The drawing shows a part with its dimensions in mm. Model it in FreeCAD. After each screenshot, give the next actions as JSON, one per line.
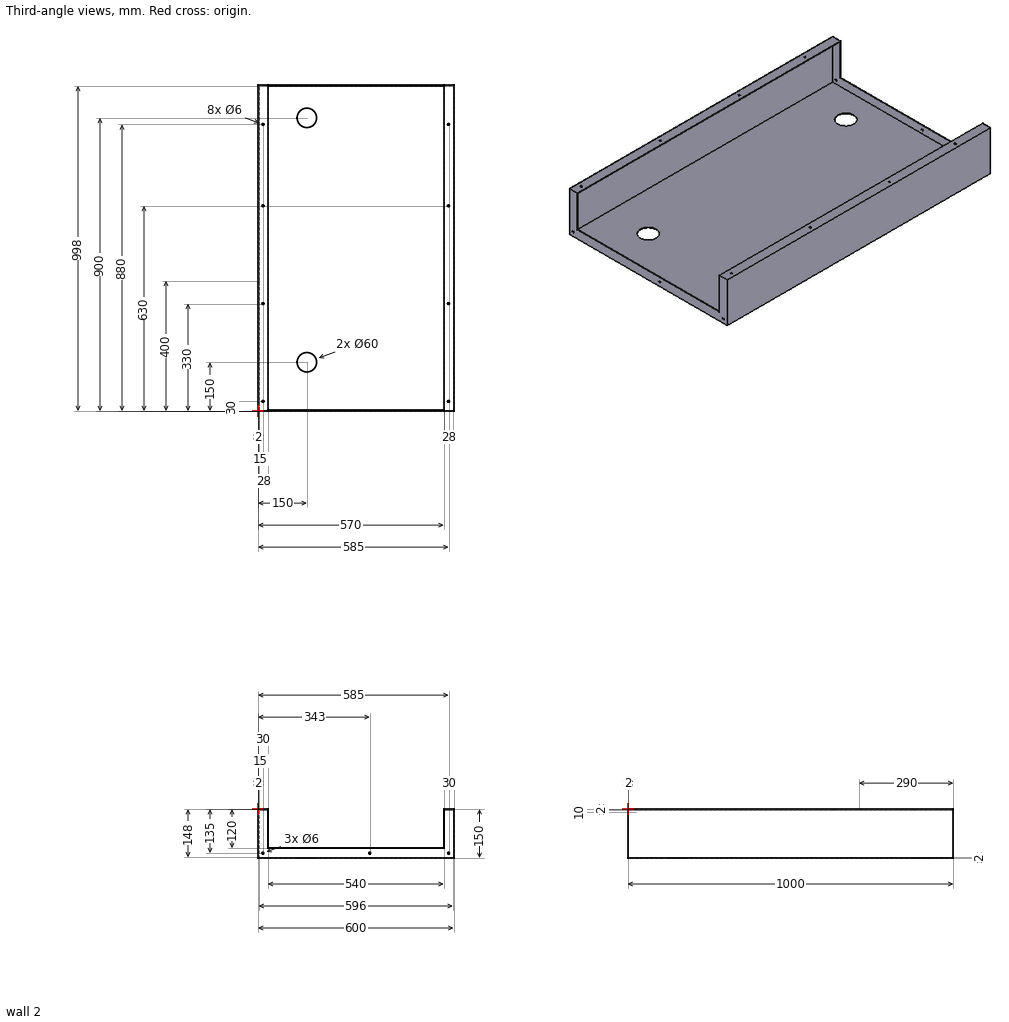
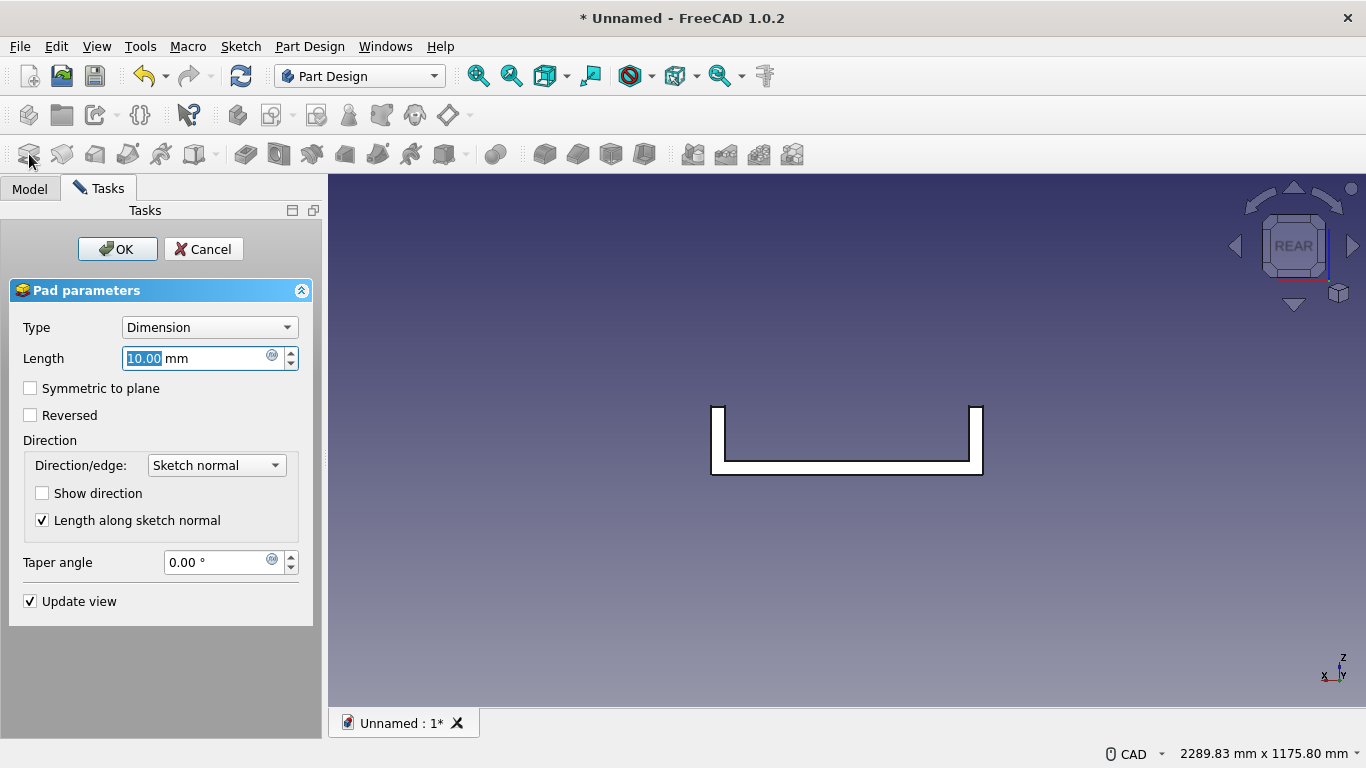
{"action": "type", "text": "2"}
{"action": "key", "text": "Tab"}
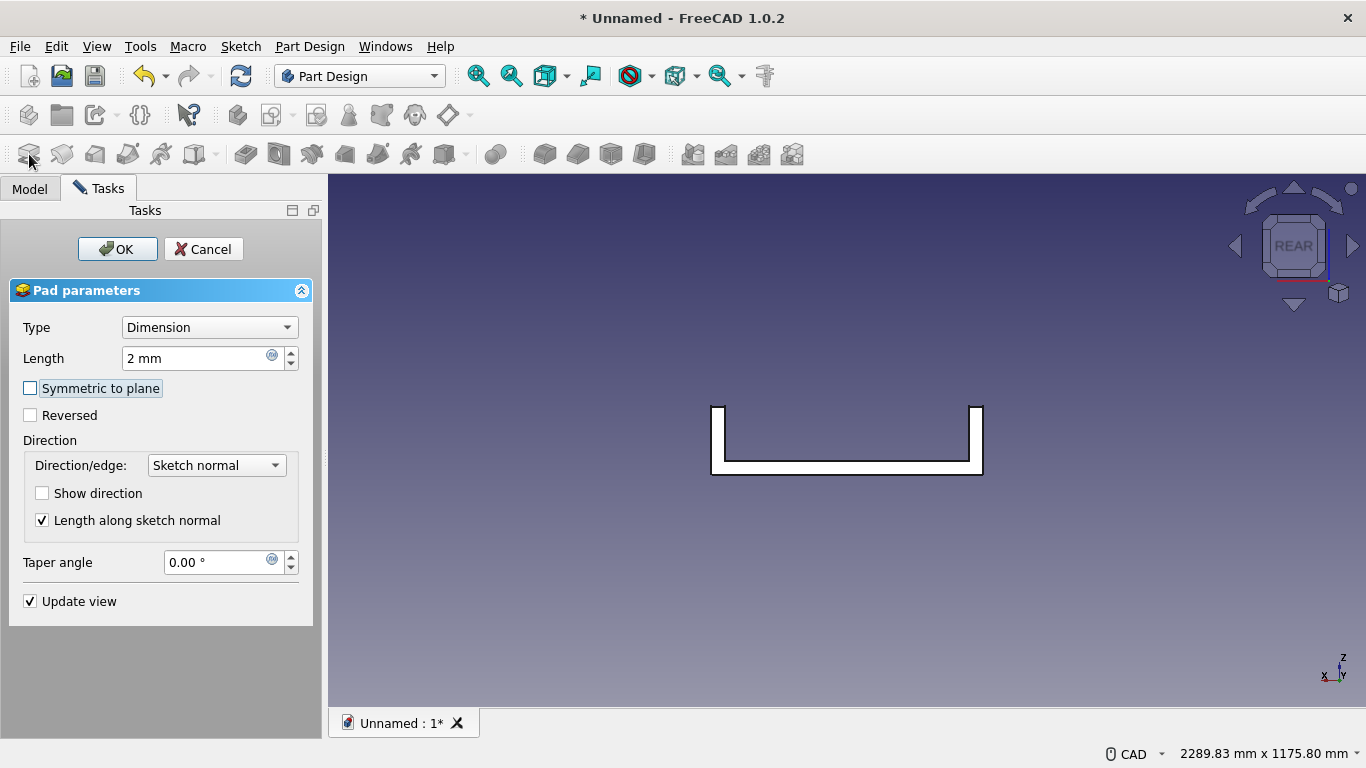
{"action": "left_click", "coordinate": [31, 415]}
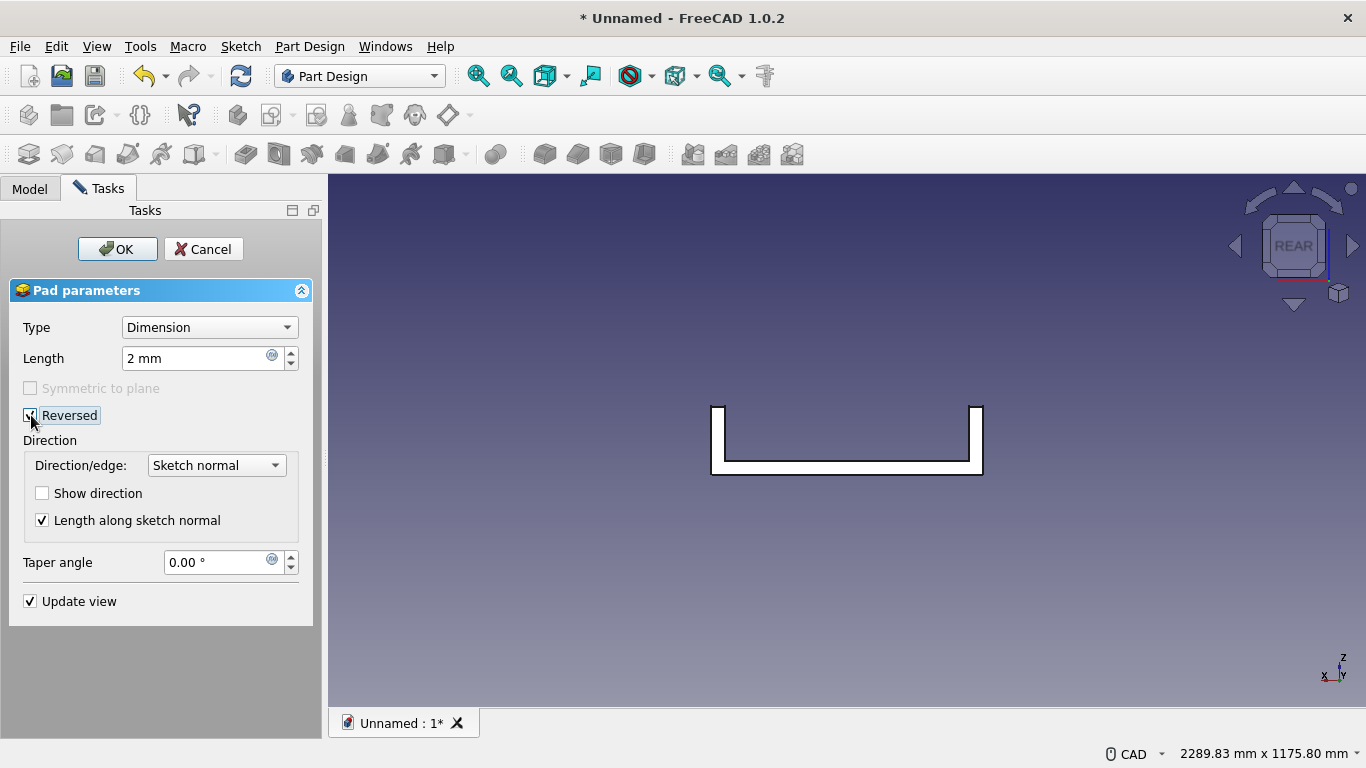
{"action": "left_click", "coordinate": [118, 249]}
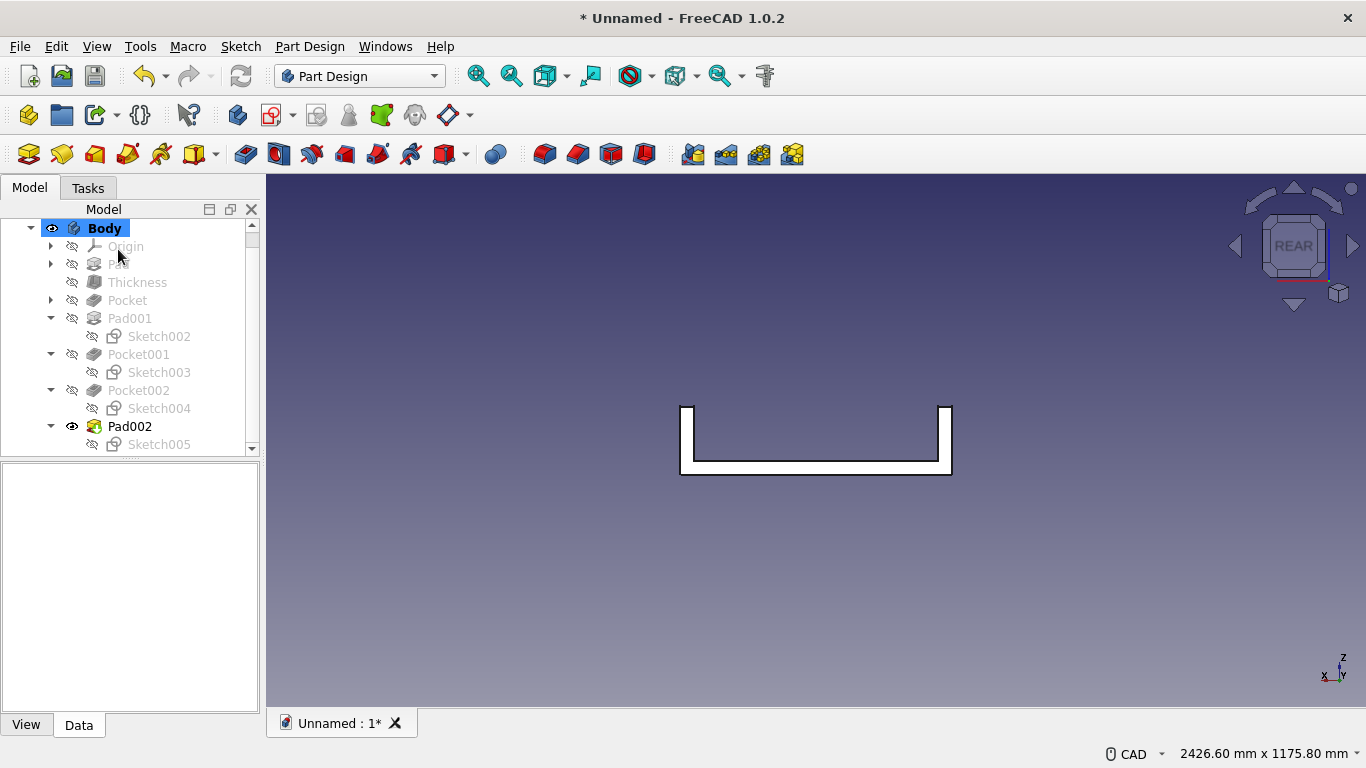
{"action": "left_click", "coordinate": [479, 76]}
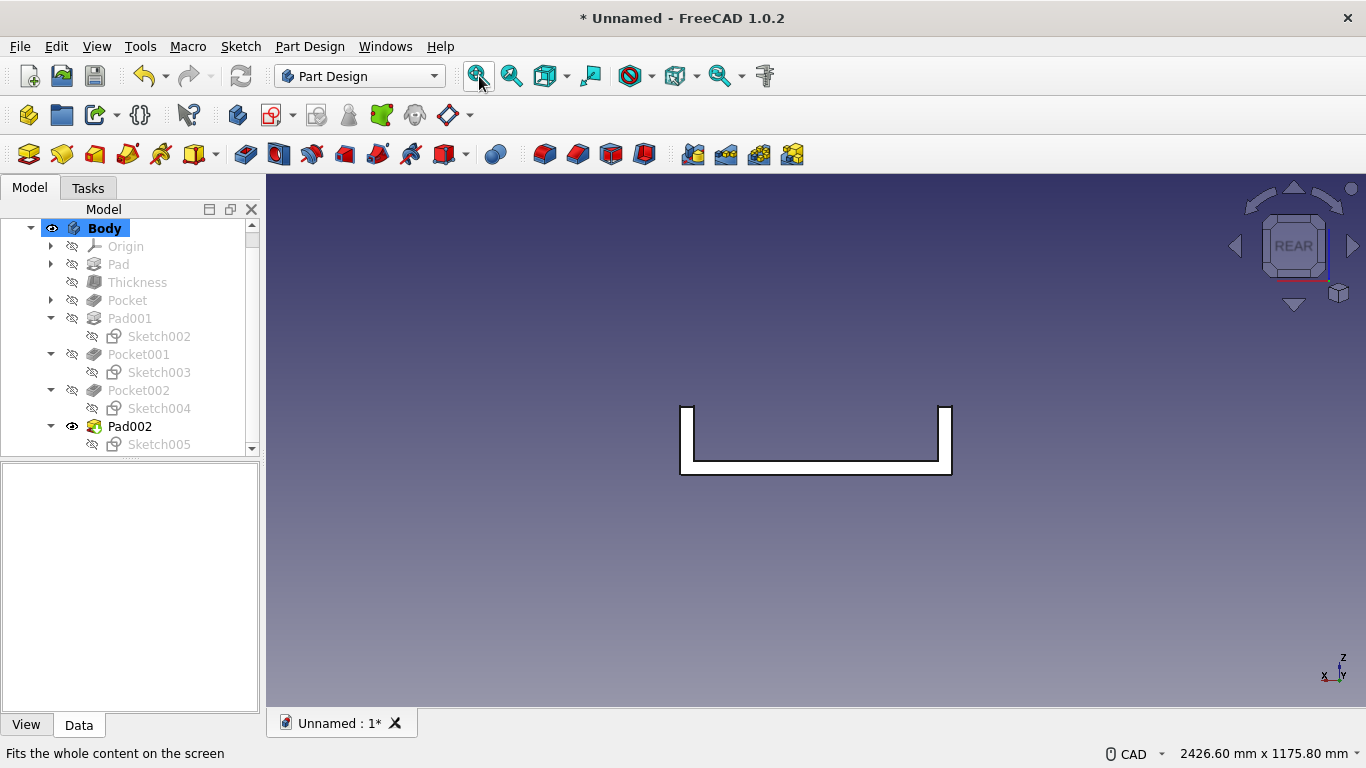
{"action": "scroll", "coordinate": [699, 469], "scroll_direction": "up", "scroll_amount": 5}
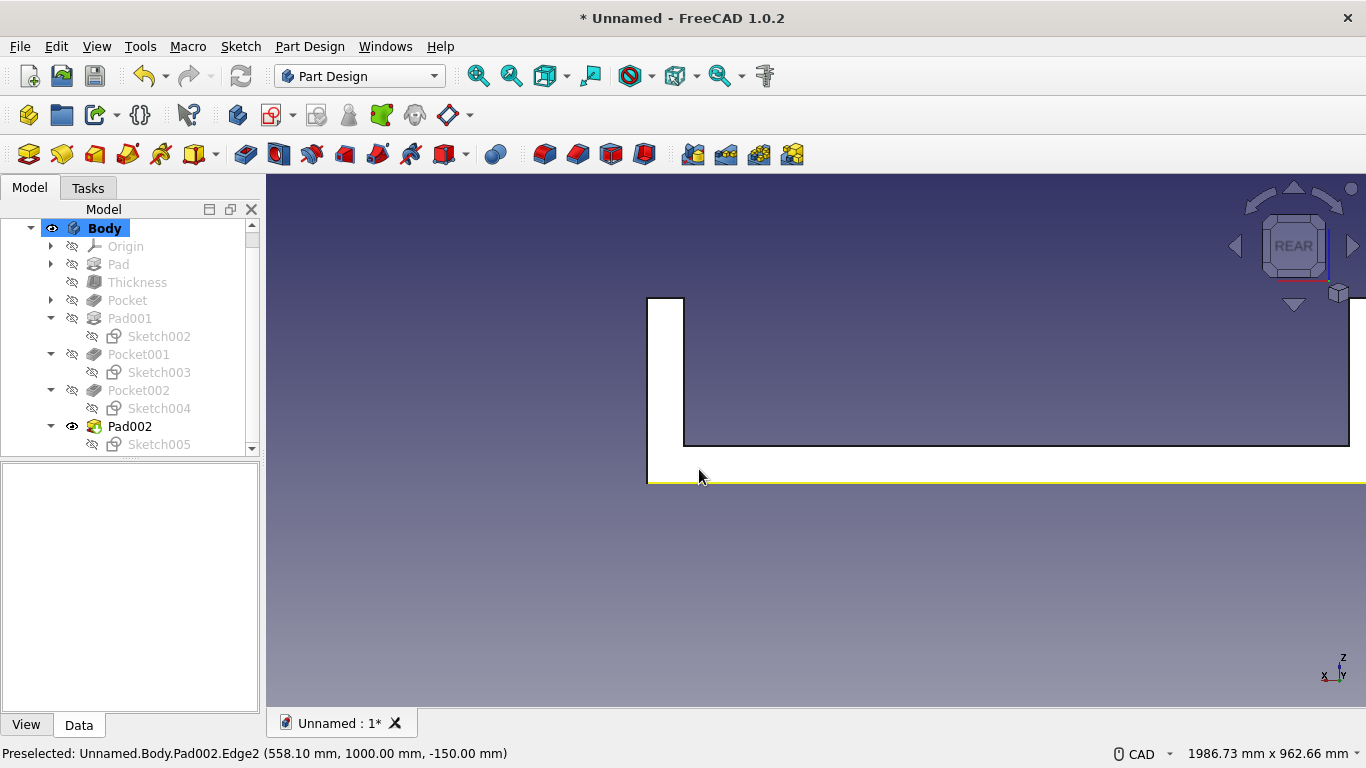
{"action": "left_click", "coordinate": [700, 469]}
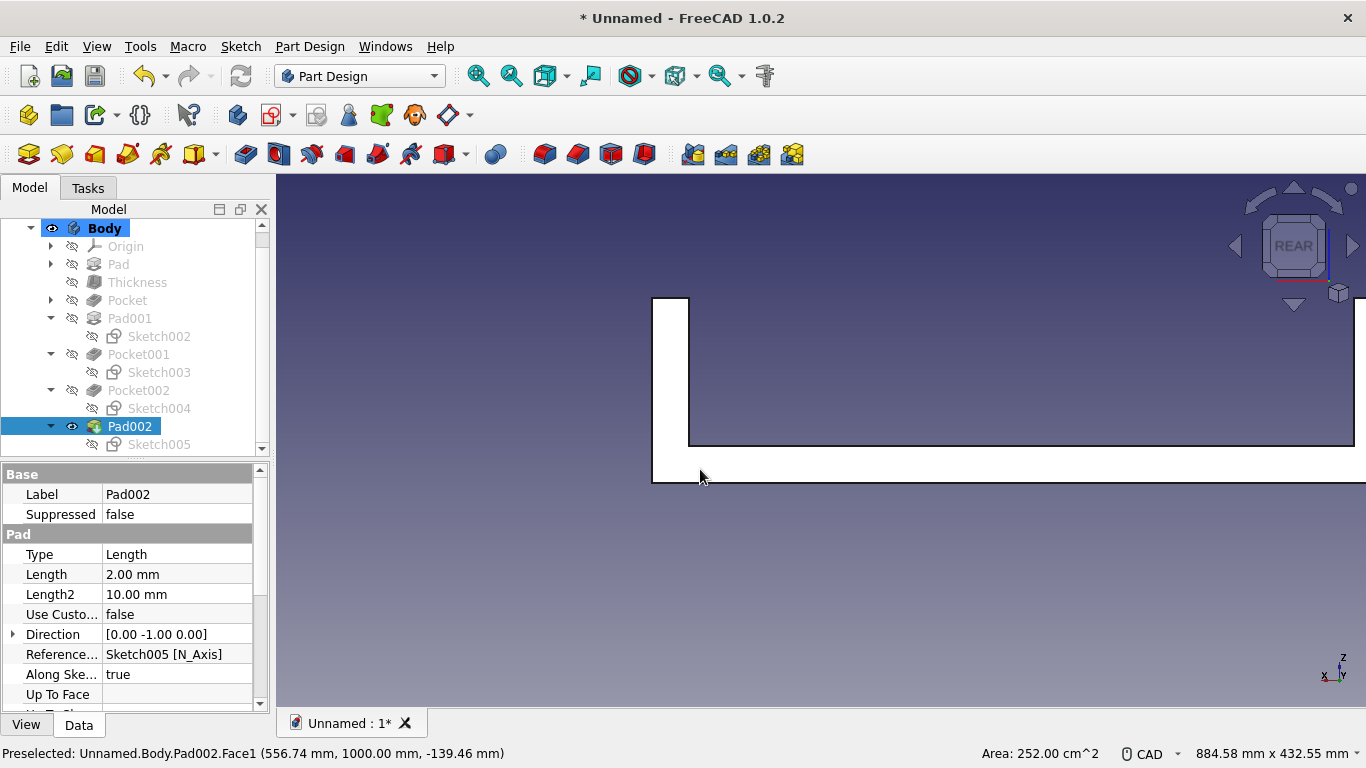
{"action": "left_click", "coordinate": [270, 116]}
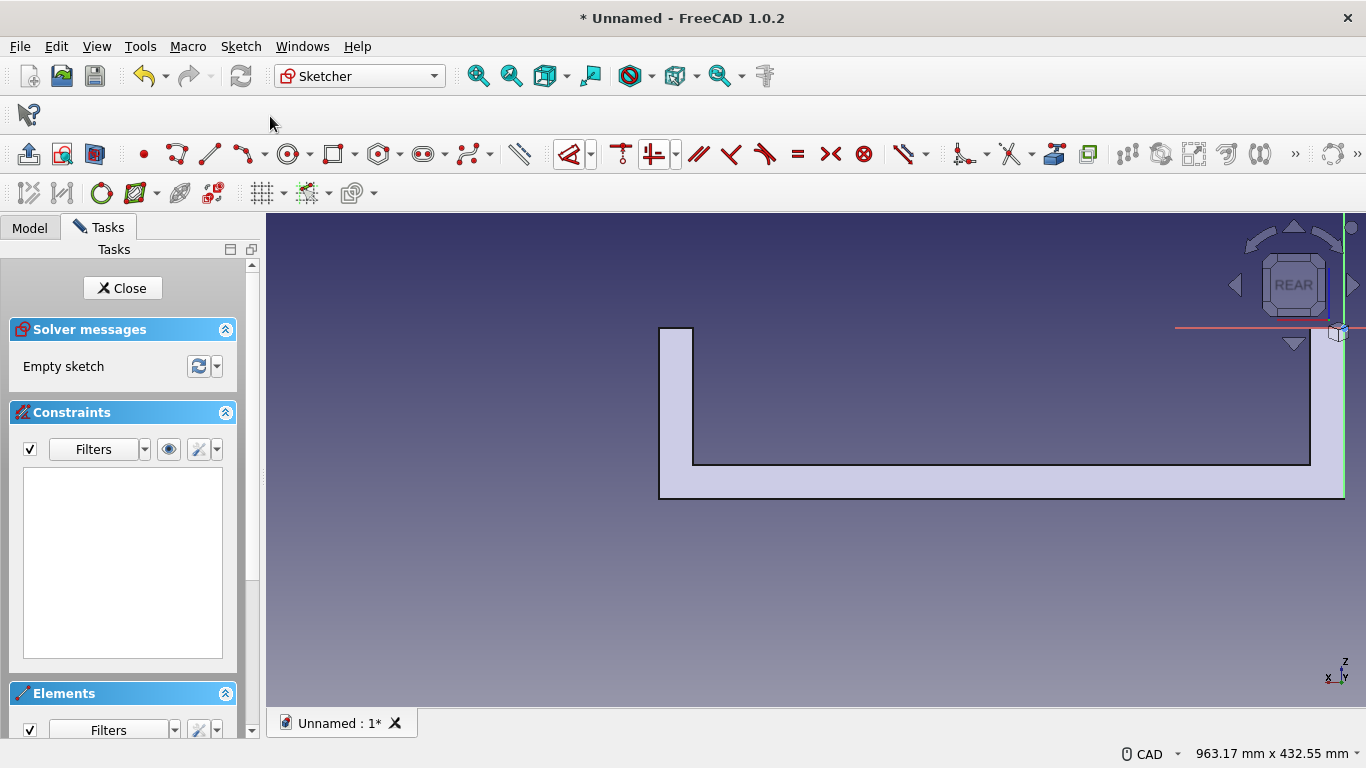
{"action": "scroll", "coordinate": [294, 679], "scroll_direction": "down", "scroll_amount": 1}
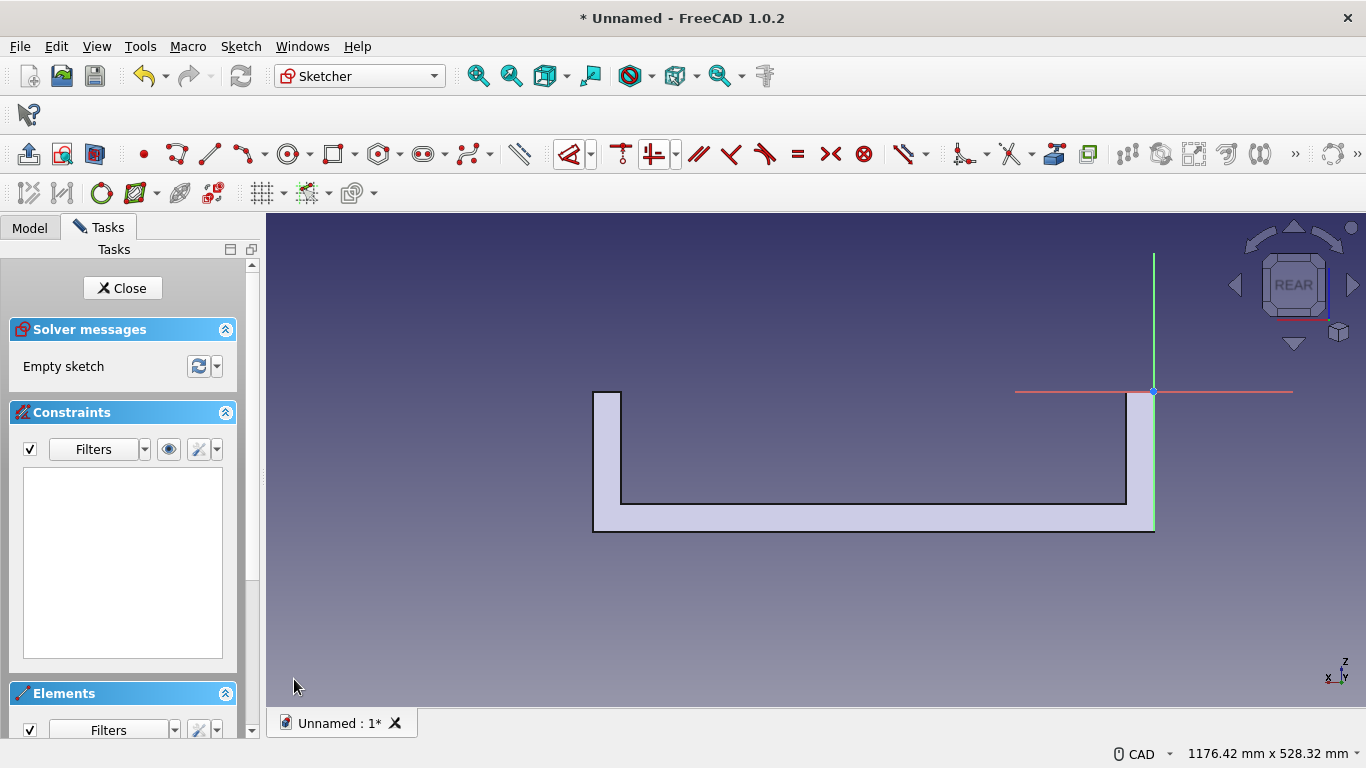
{"action": "left_click", "coordinate": [288, 154]}